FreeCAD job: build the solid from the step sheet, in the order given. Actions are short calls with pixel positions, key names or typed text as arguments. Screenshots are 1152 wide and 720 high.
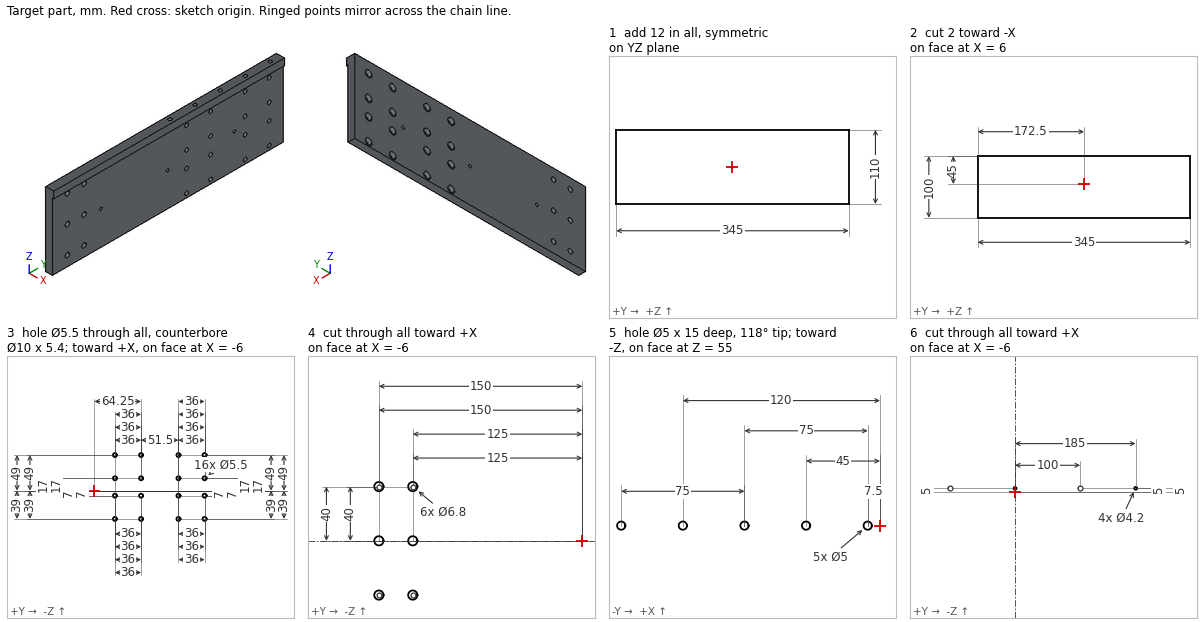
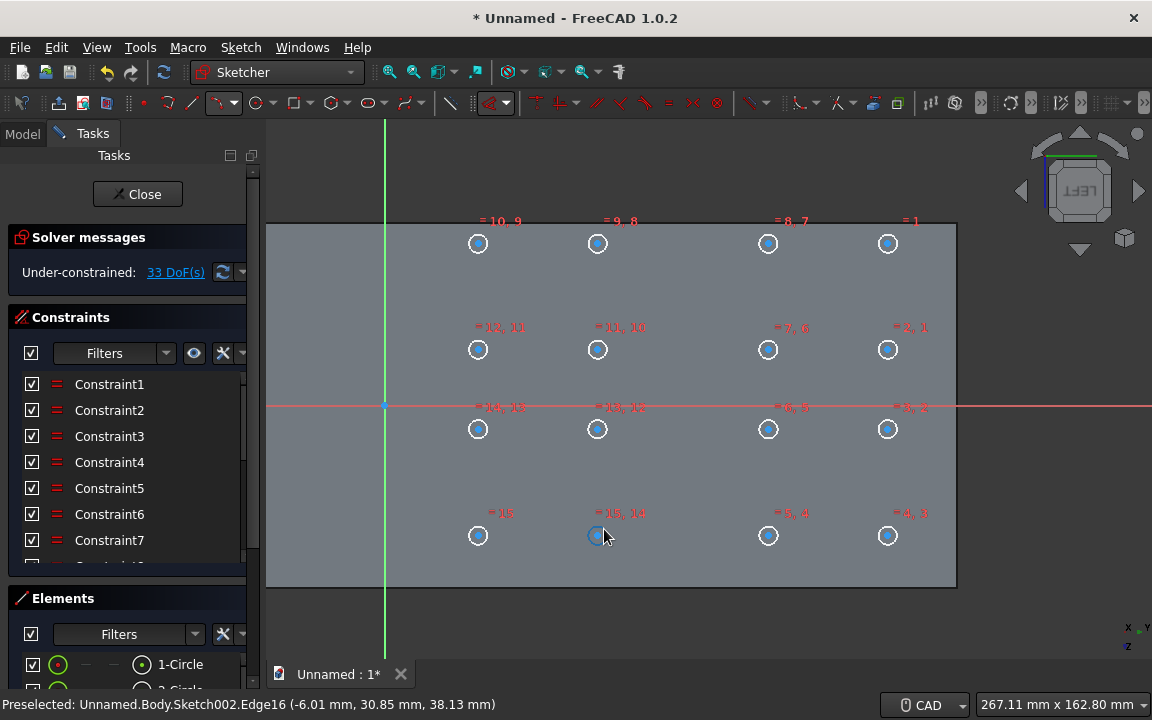
scroll(894, 237, up, 4)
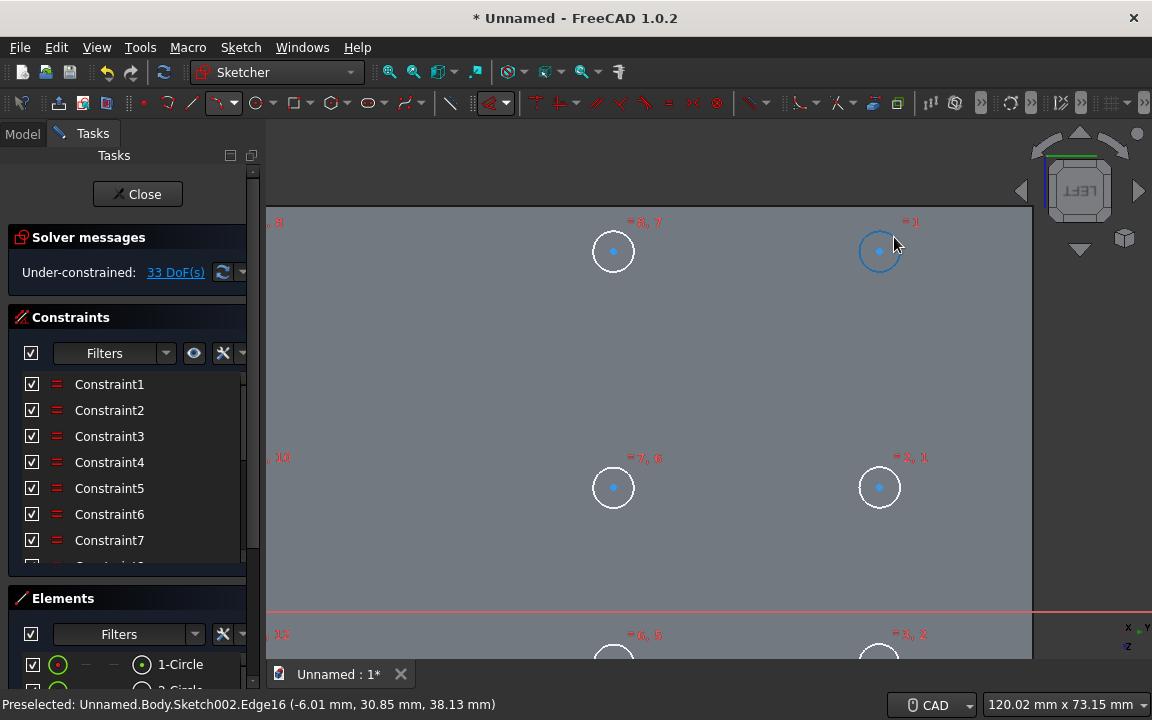
click(894, 237)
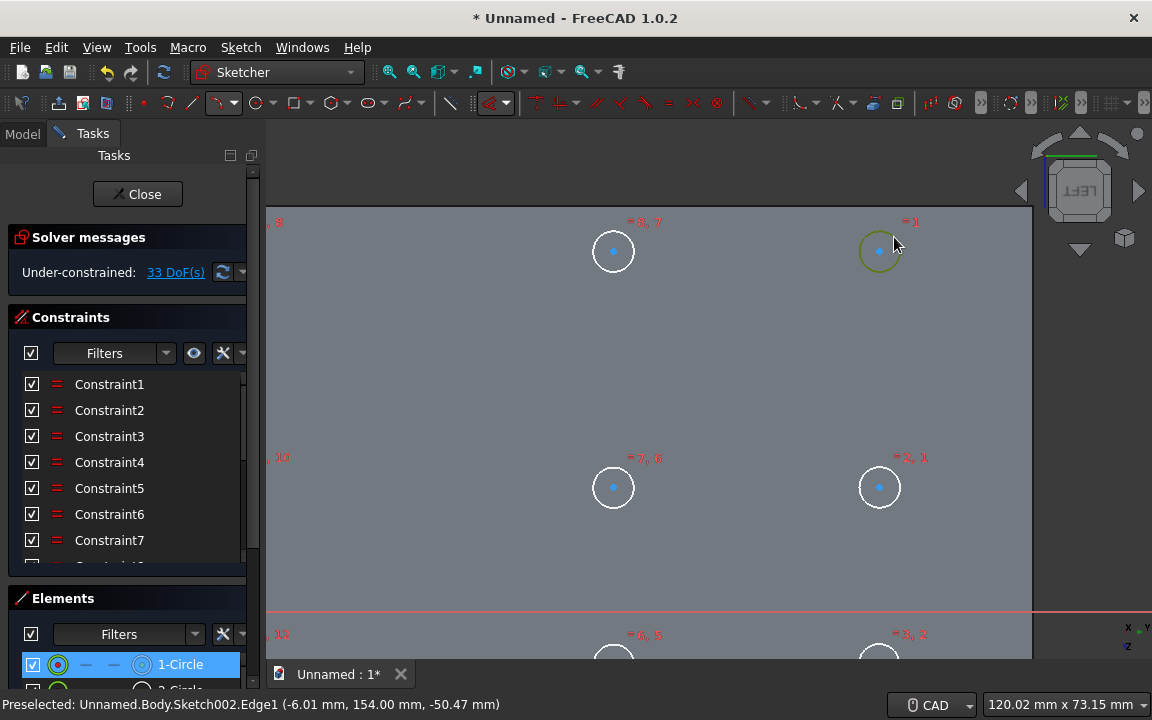
click(508, 104)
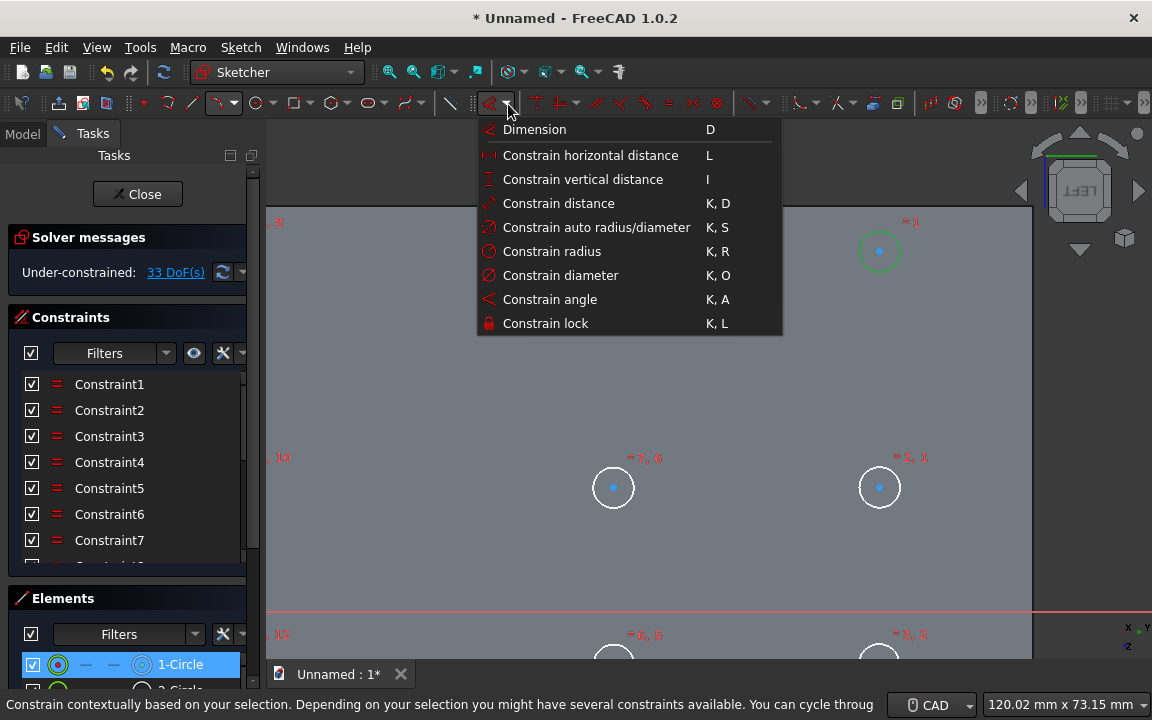
click(630, 275)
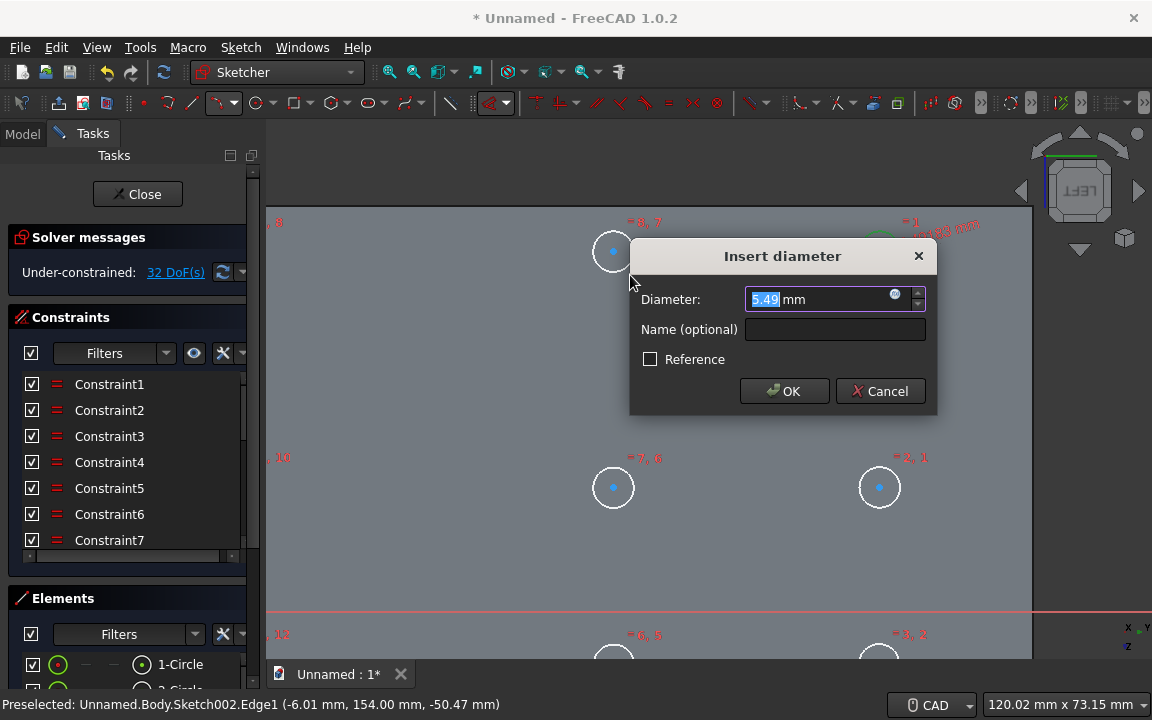
text(5.5)
key(Return)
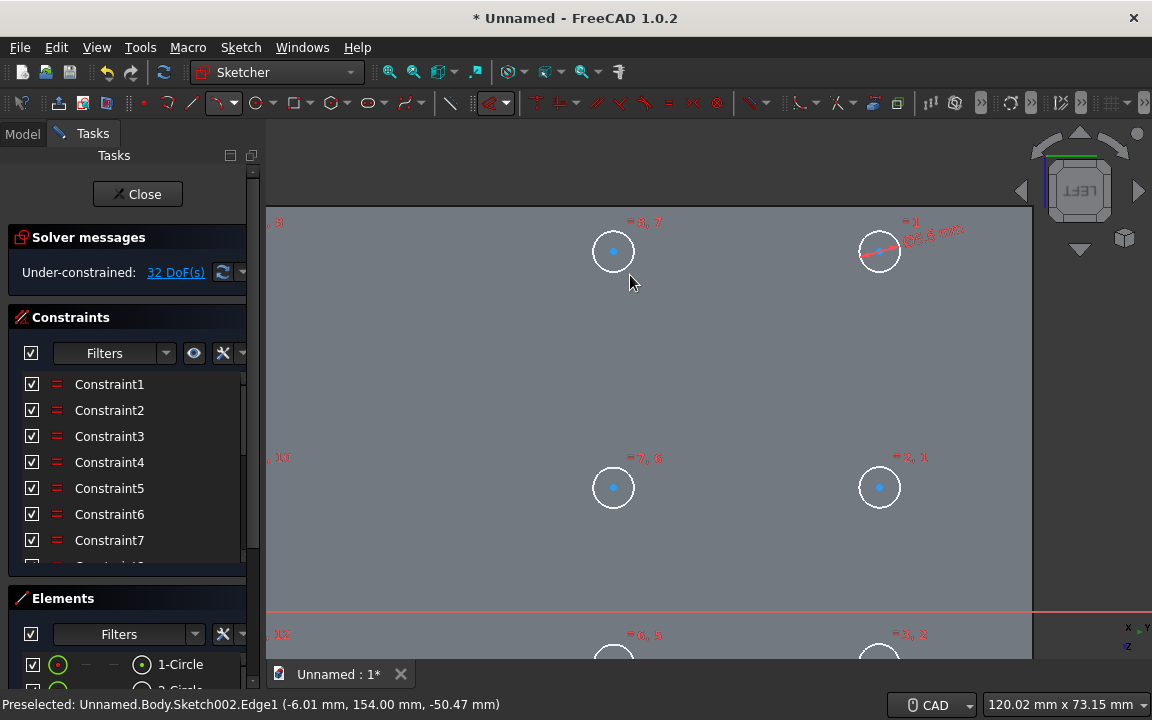
scroll(894, 237, down, 4)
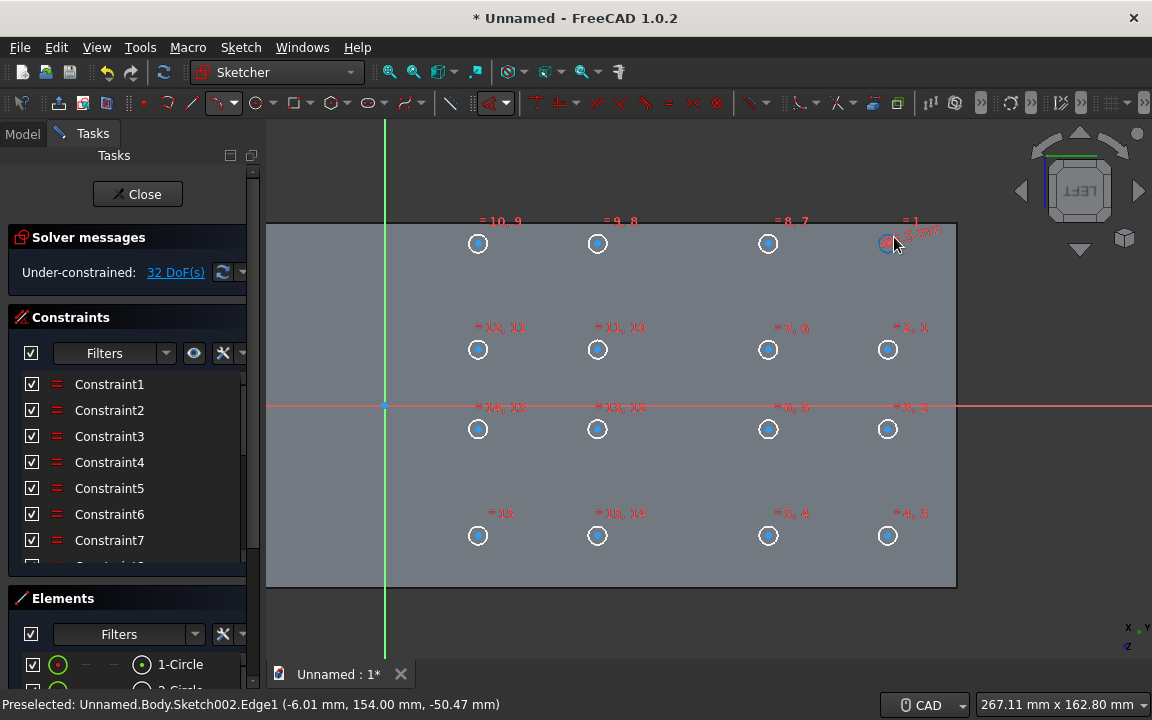
scroll(888, 429, up, 3)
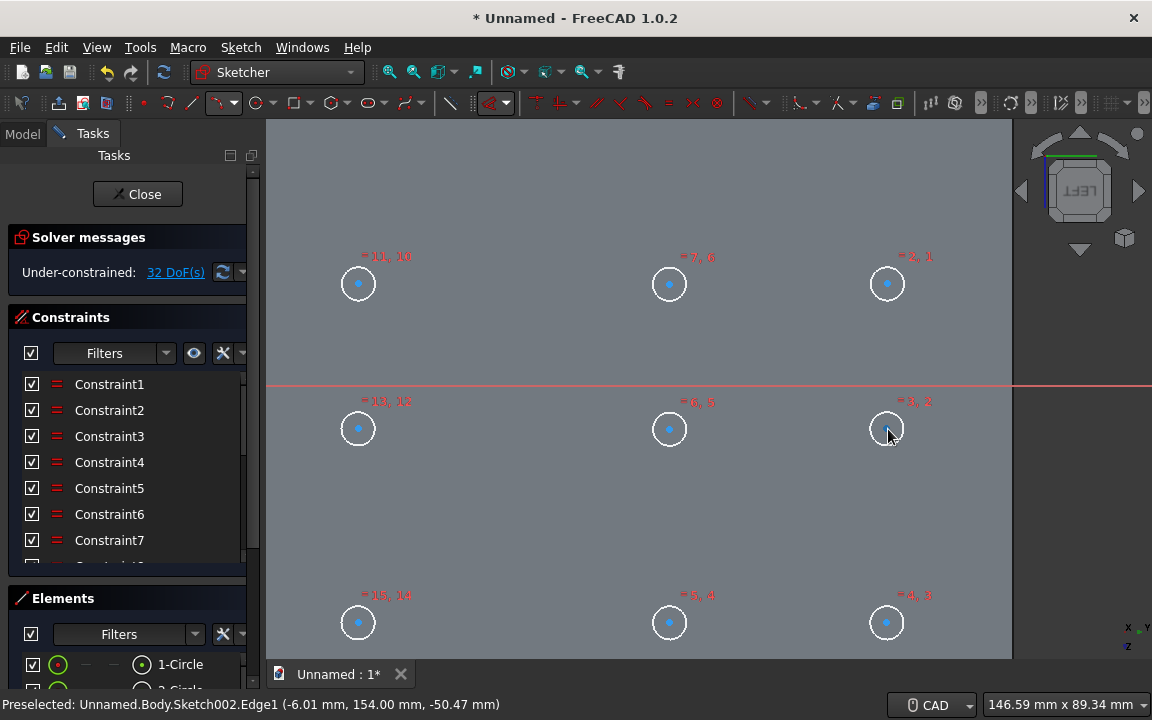
click(887, 429)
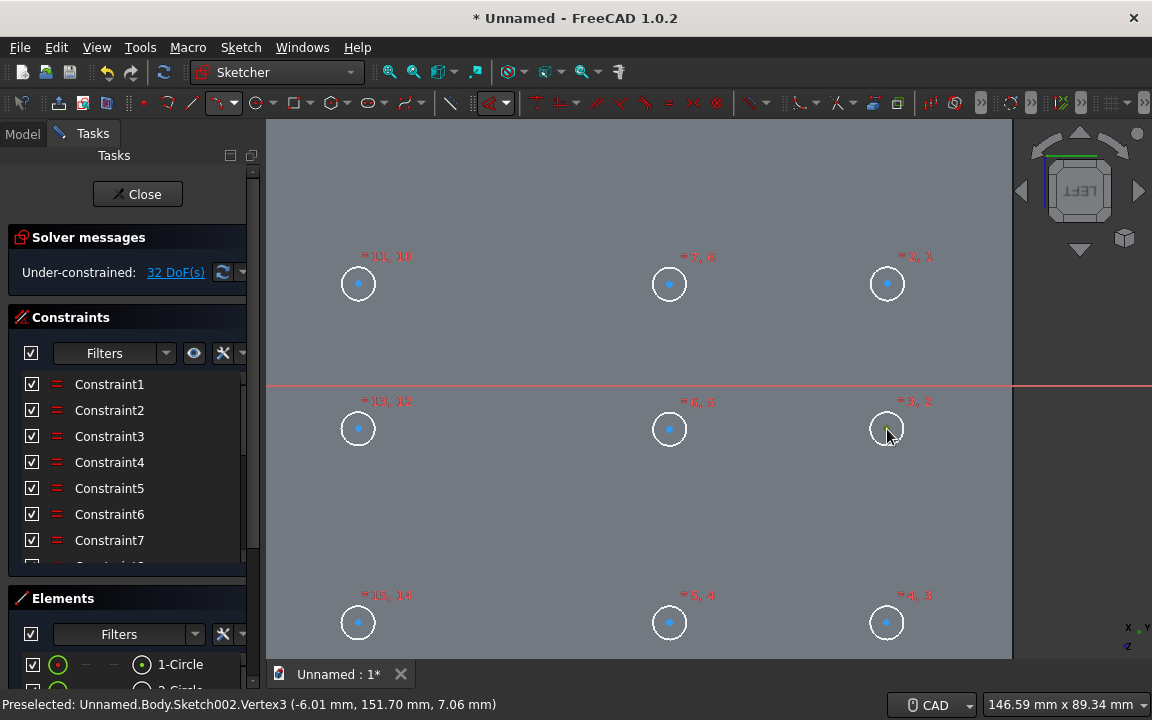
click(508, 104)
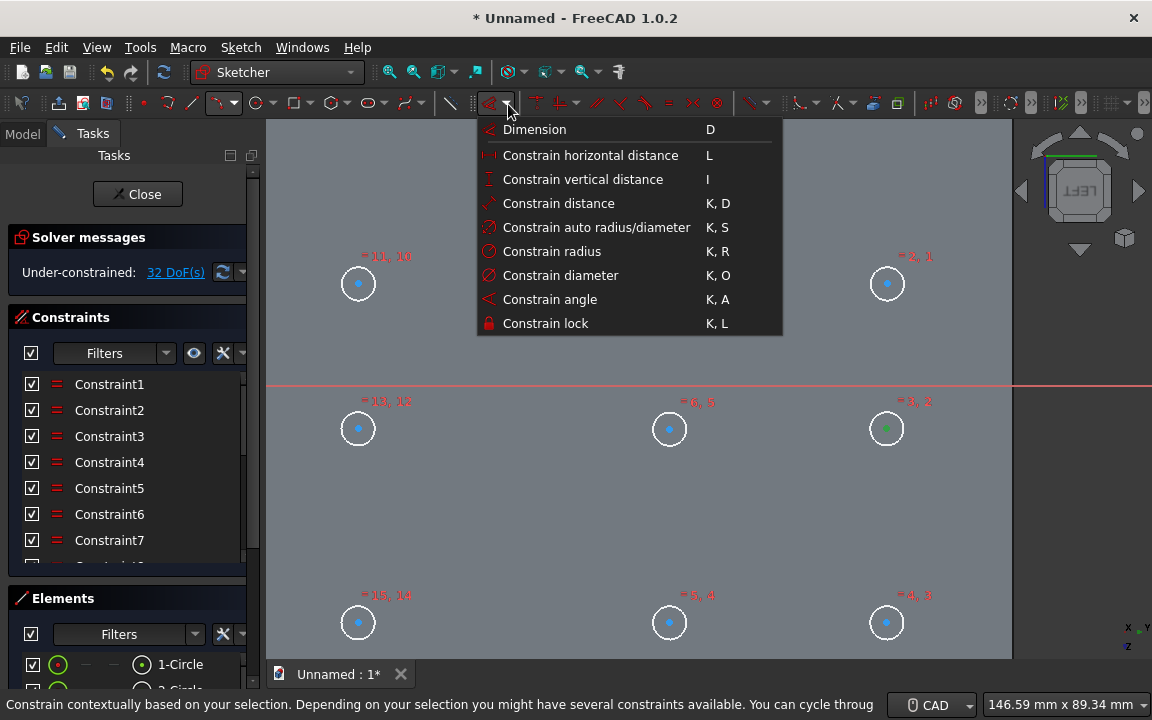
click(630, 179)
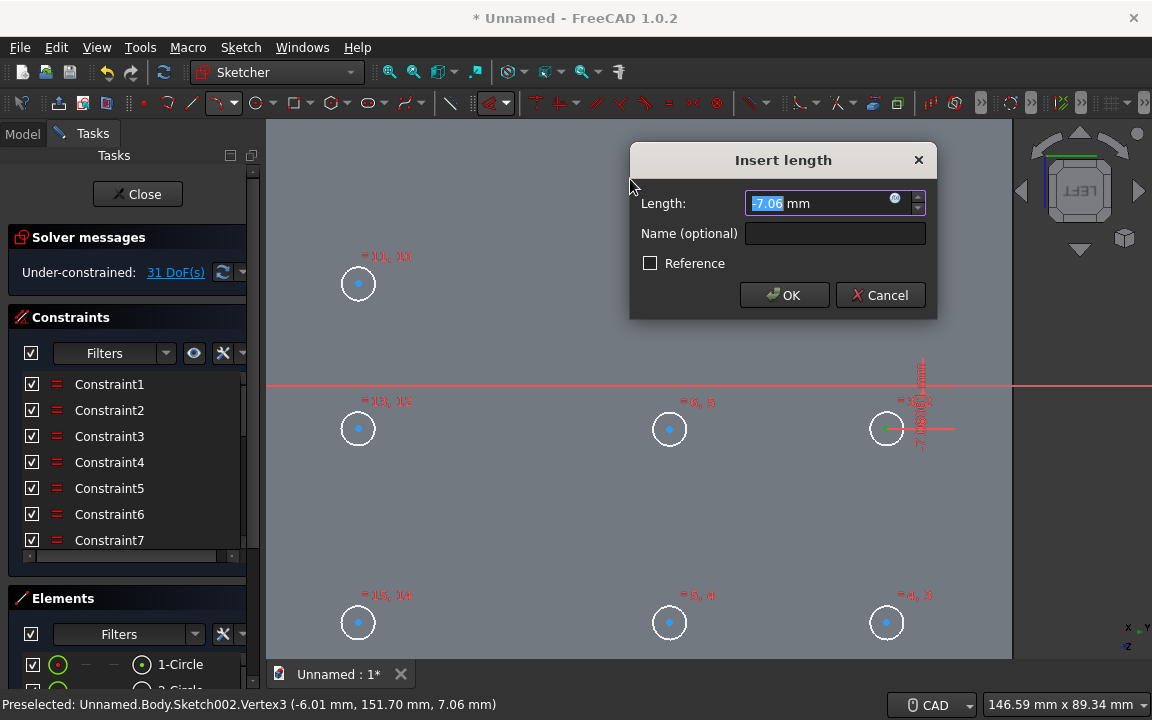
text(-7)
key(Return)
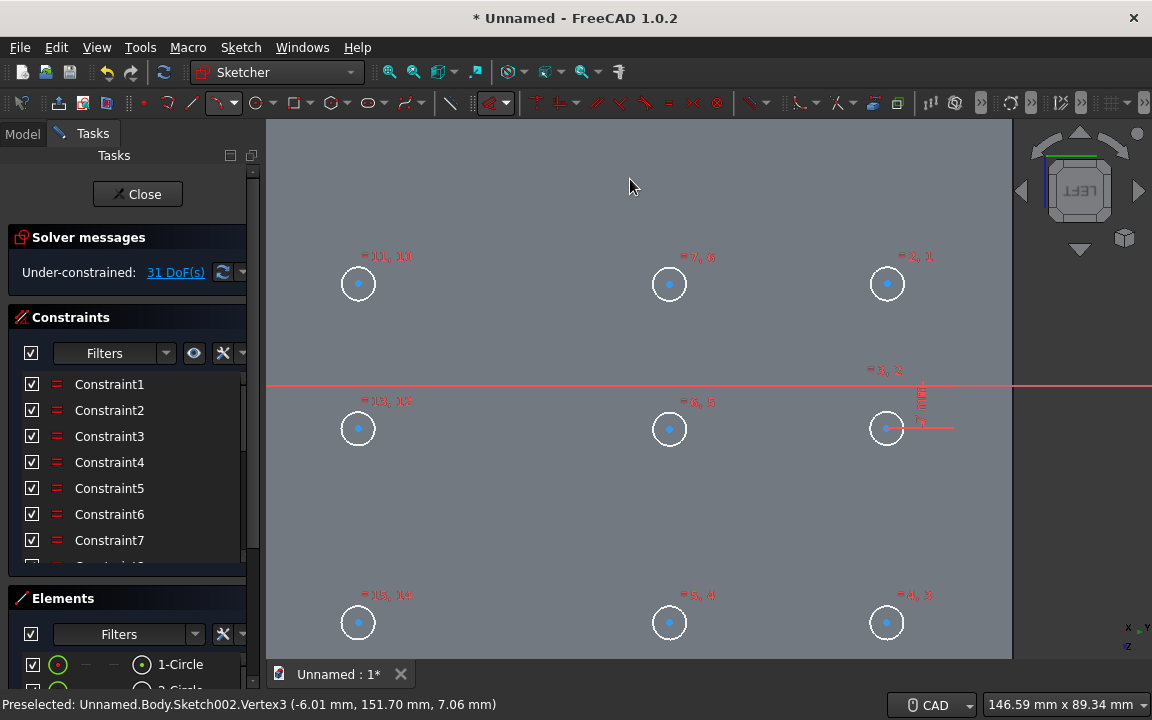
click(670, 429)